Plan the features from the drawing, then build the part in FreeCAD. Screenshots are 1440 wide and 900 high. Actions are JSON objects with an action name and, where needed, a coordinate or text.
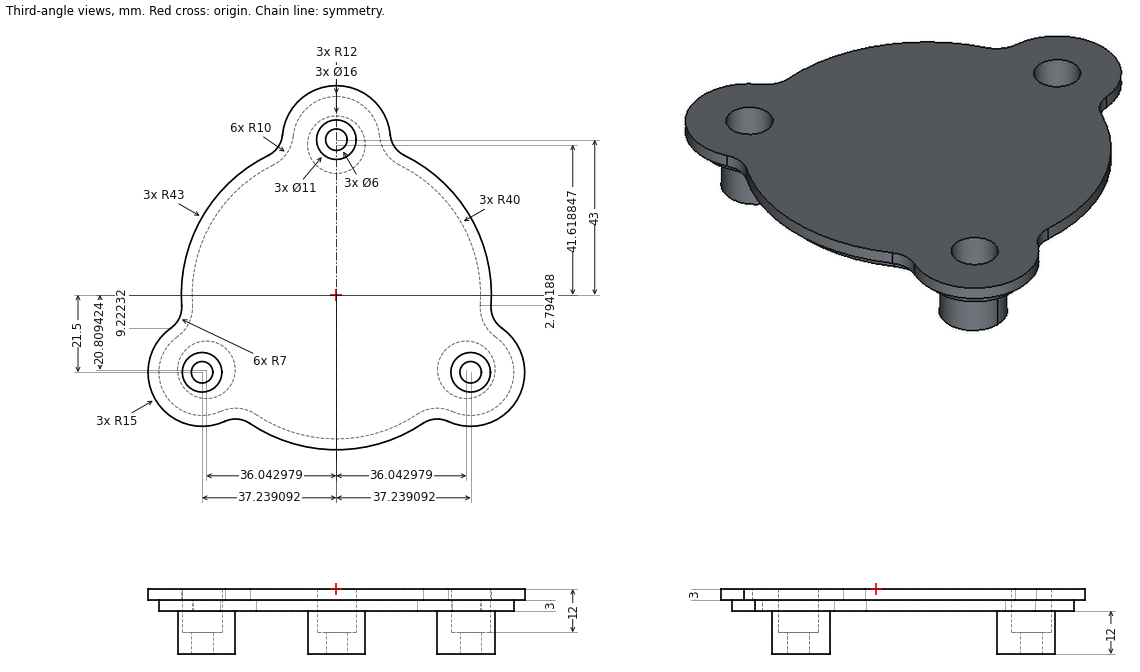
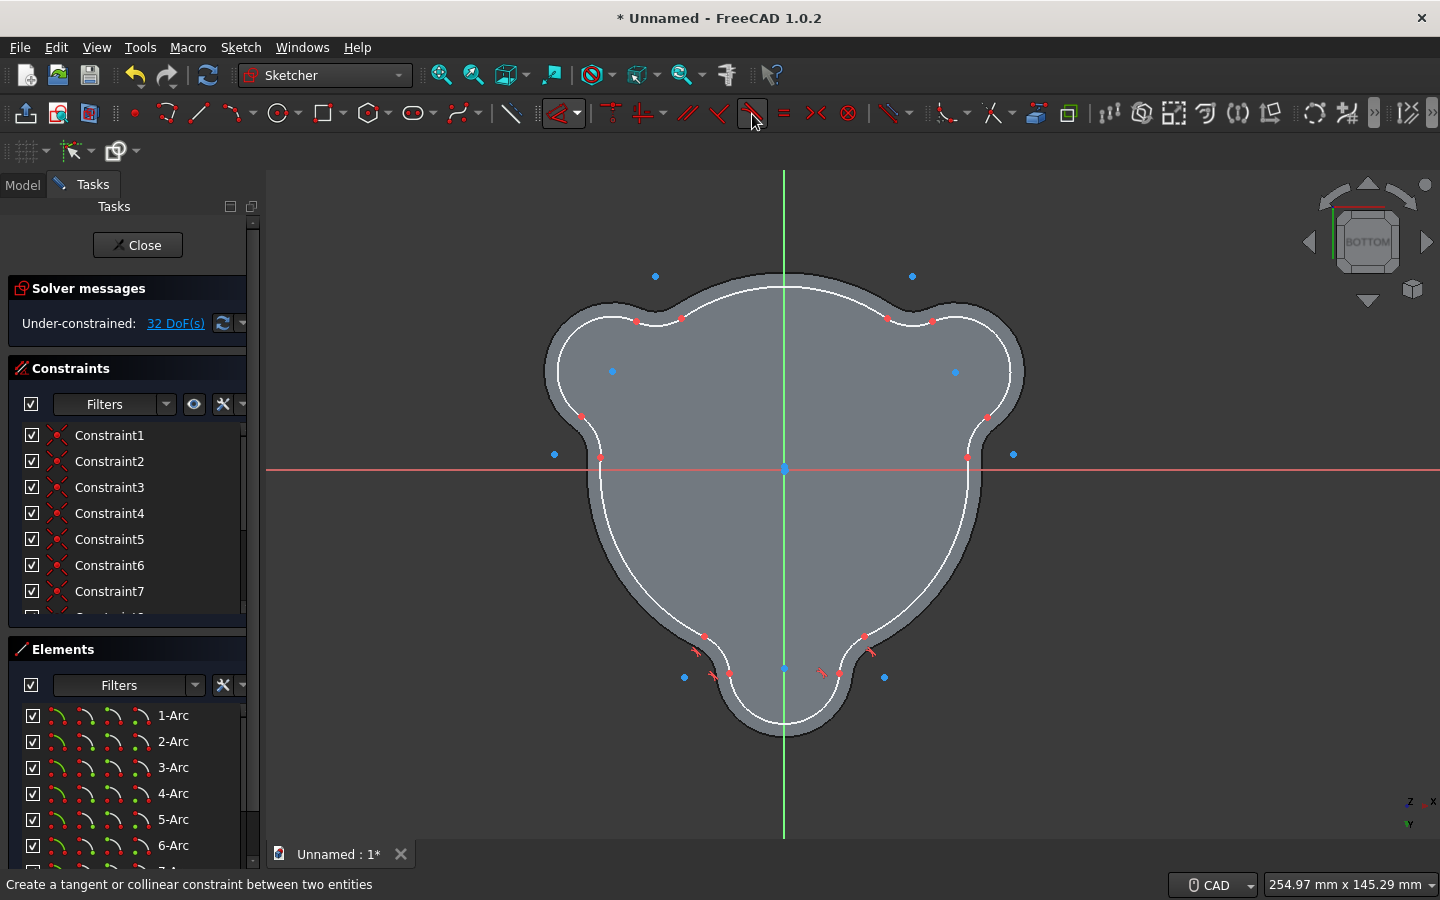
{"action": "left_click", "coordinate": [918, 598]}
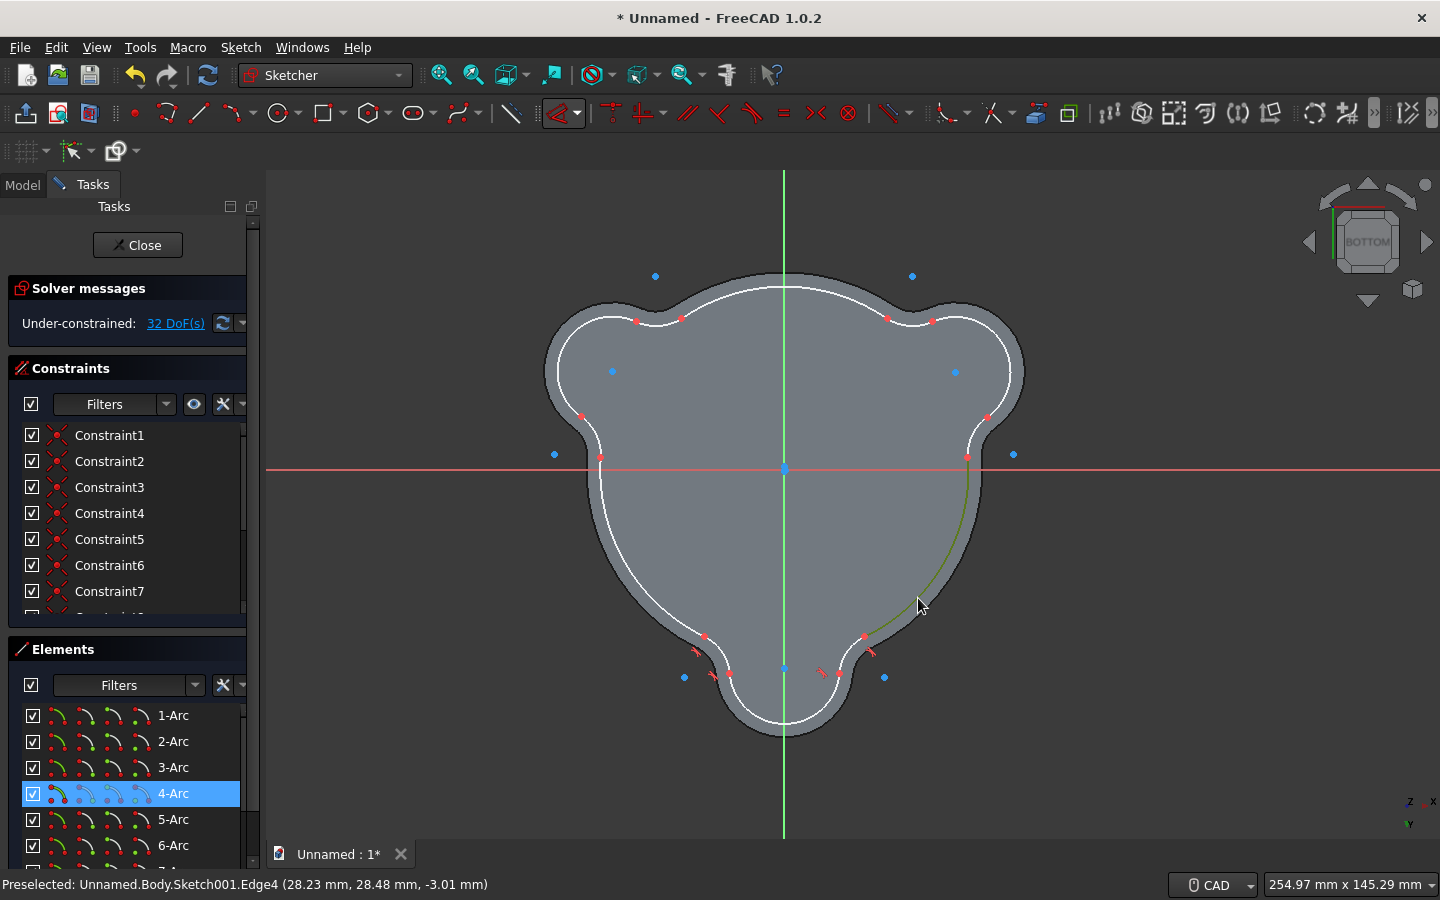
{"action": "left_click", "coordinate": [977, 427]}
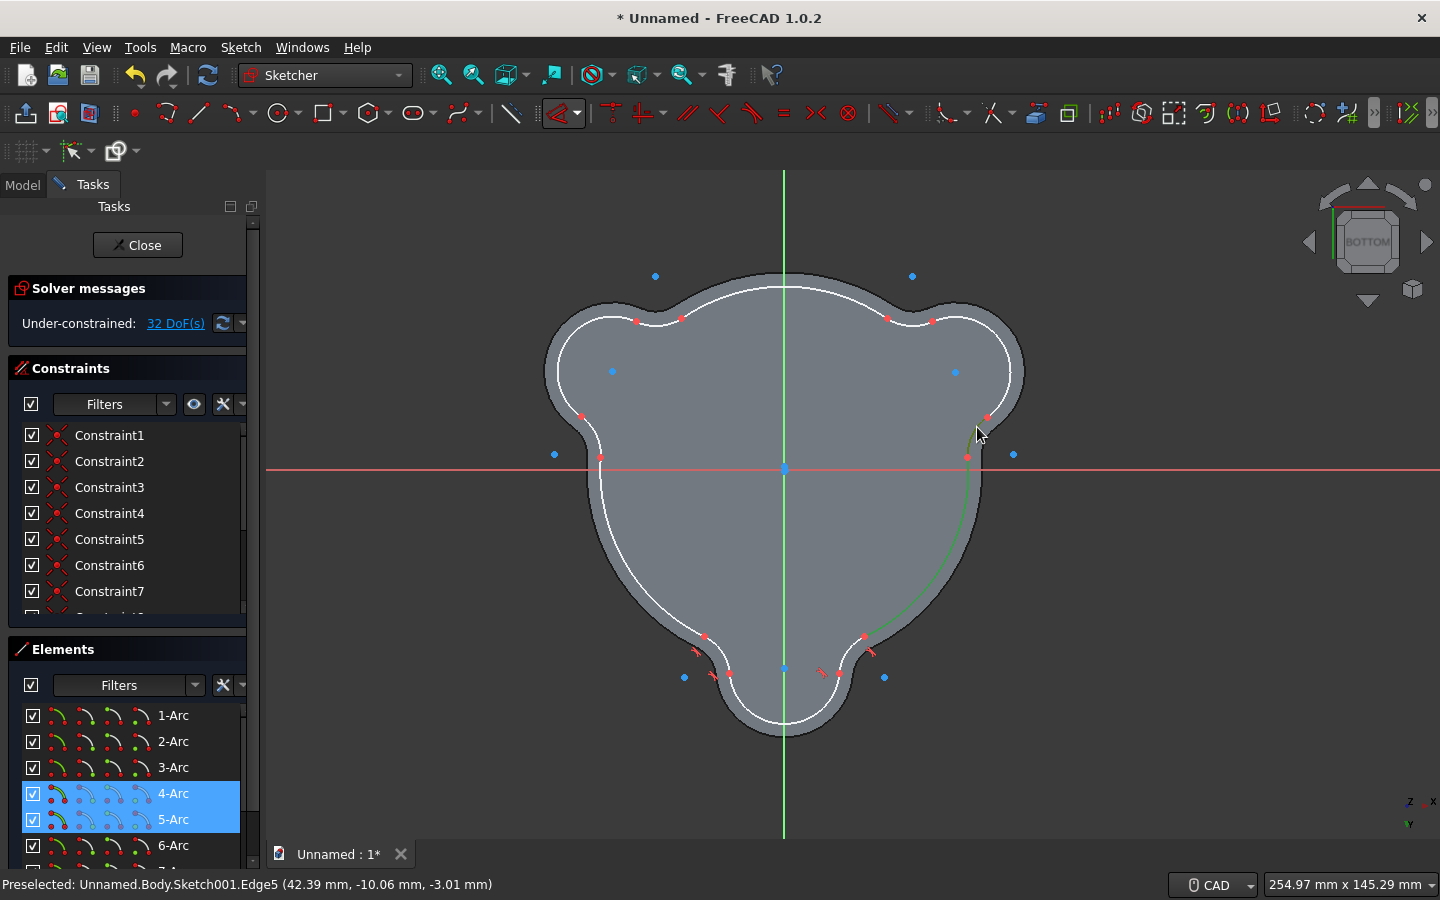
{"action": "left_click", "coordinate": [752, 114]}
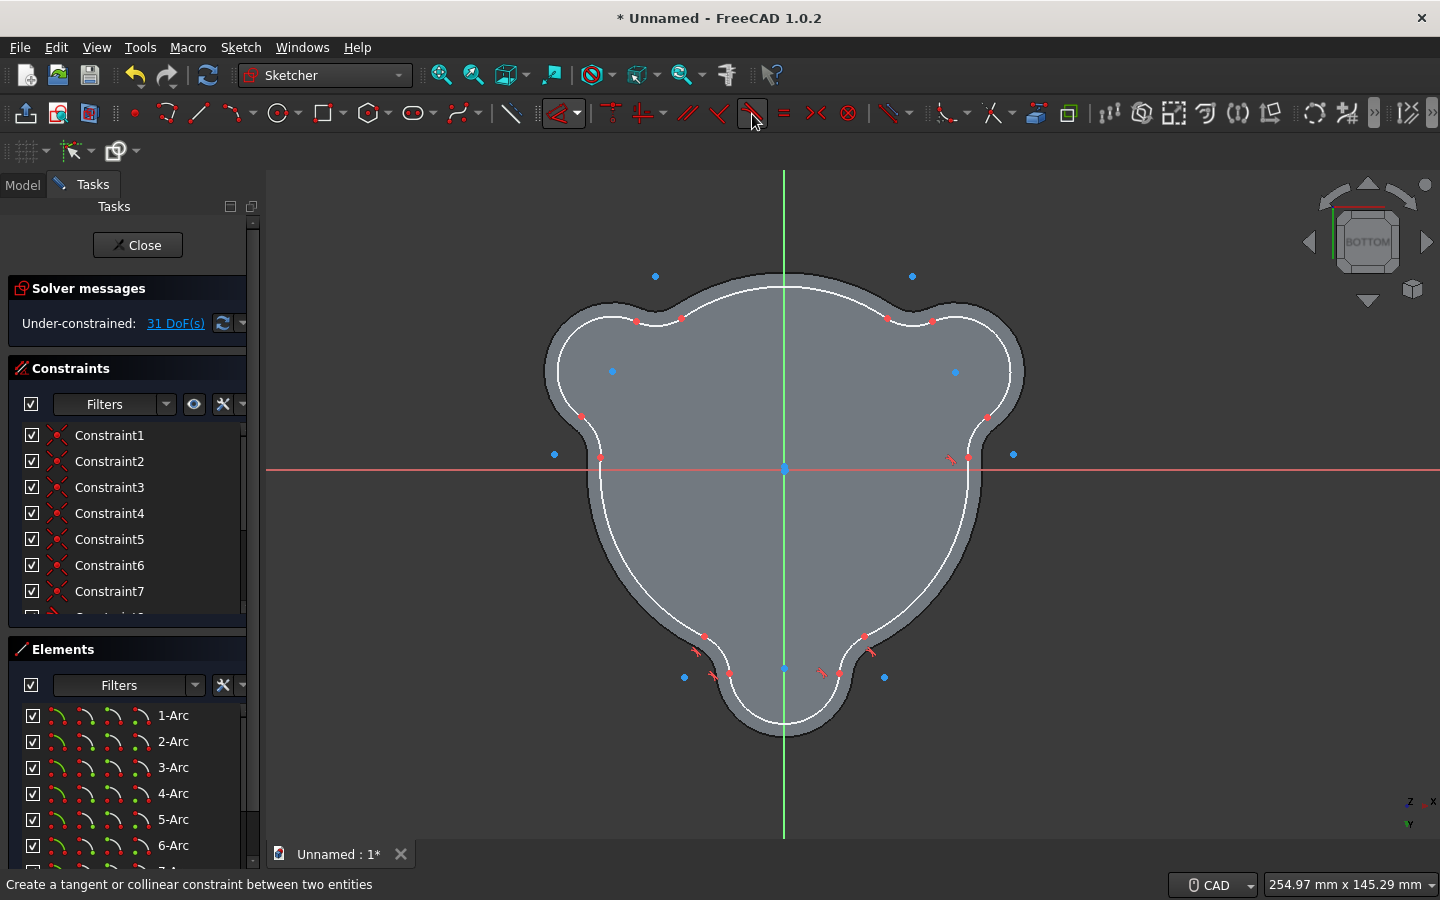
{"action": "left_click", "coordinate": [977, 427]}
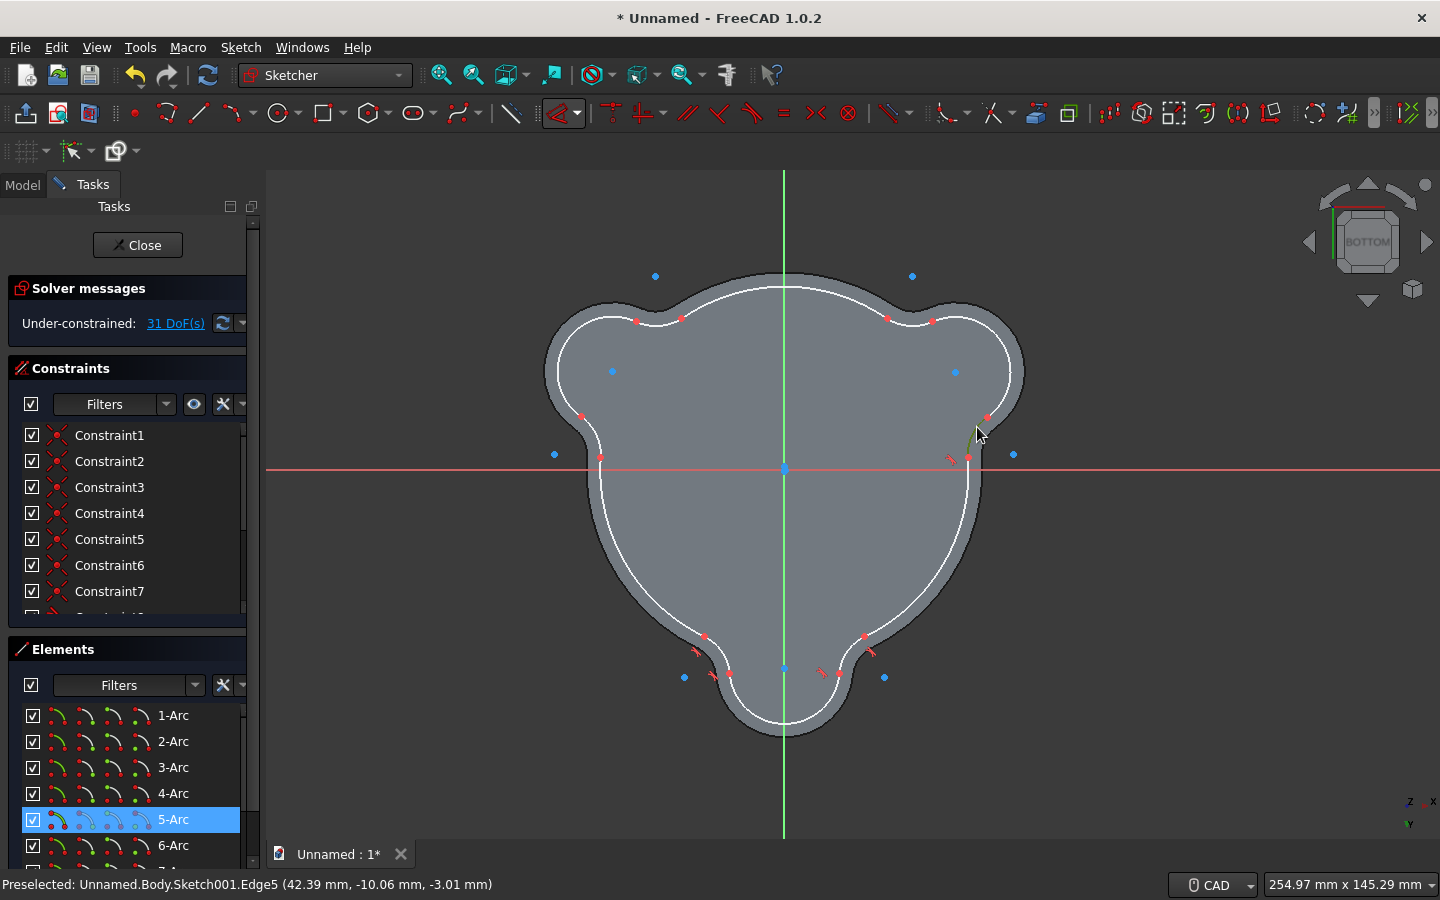
{"action": "left_click", "coordinate": [1010, 376]}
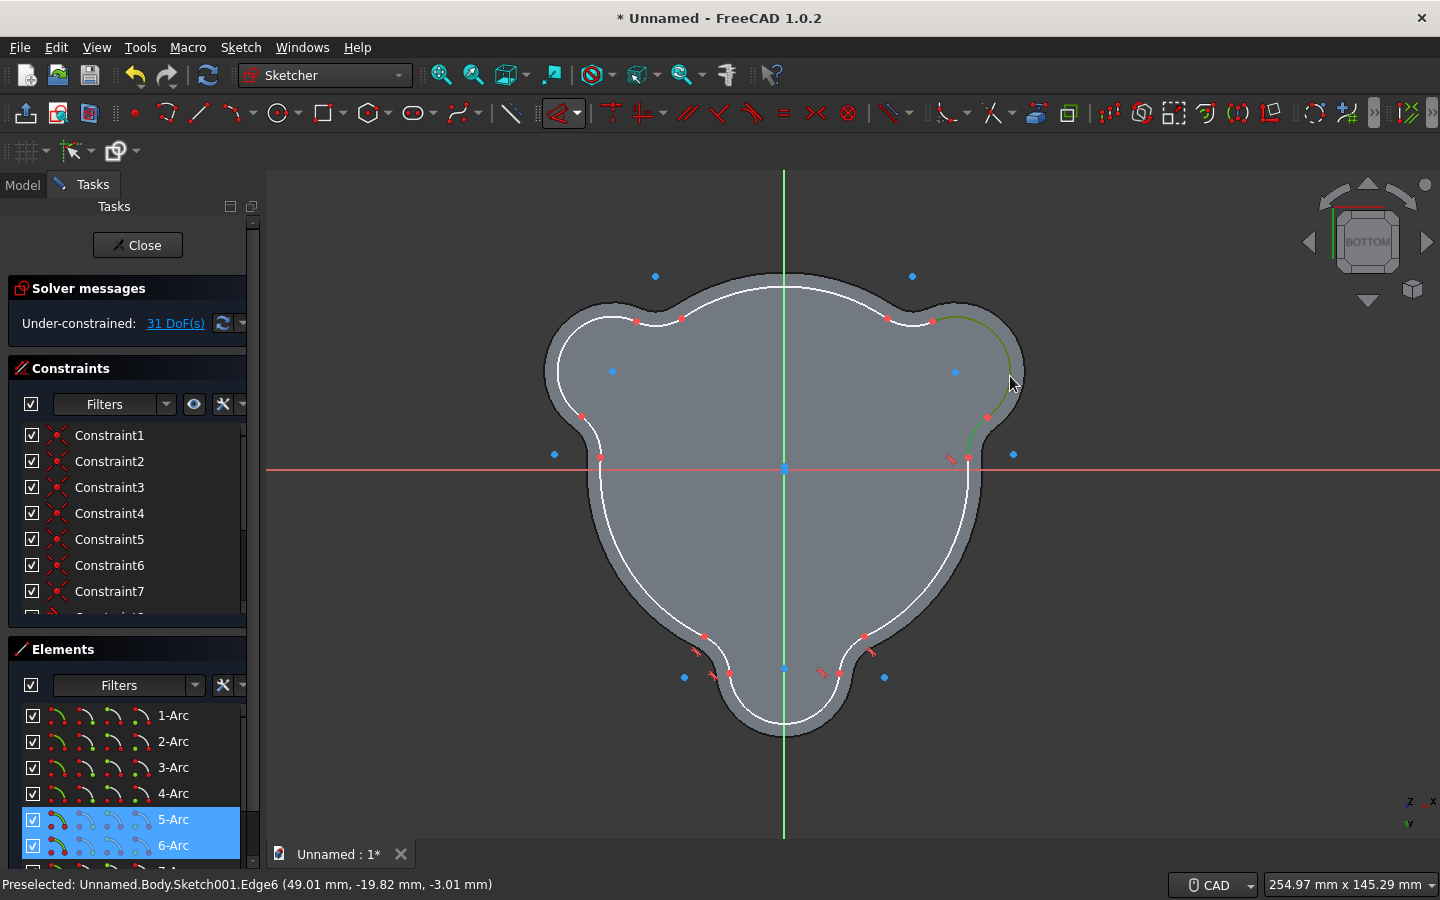
{"action": "left_click", "coordinate": [752, 114]}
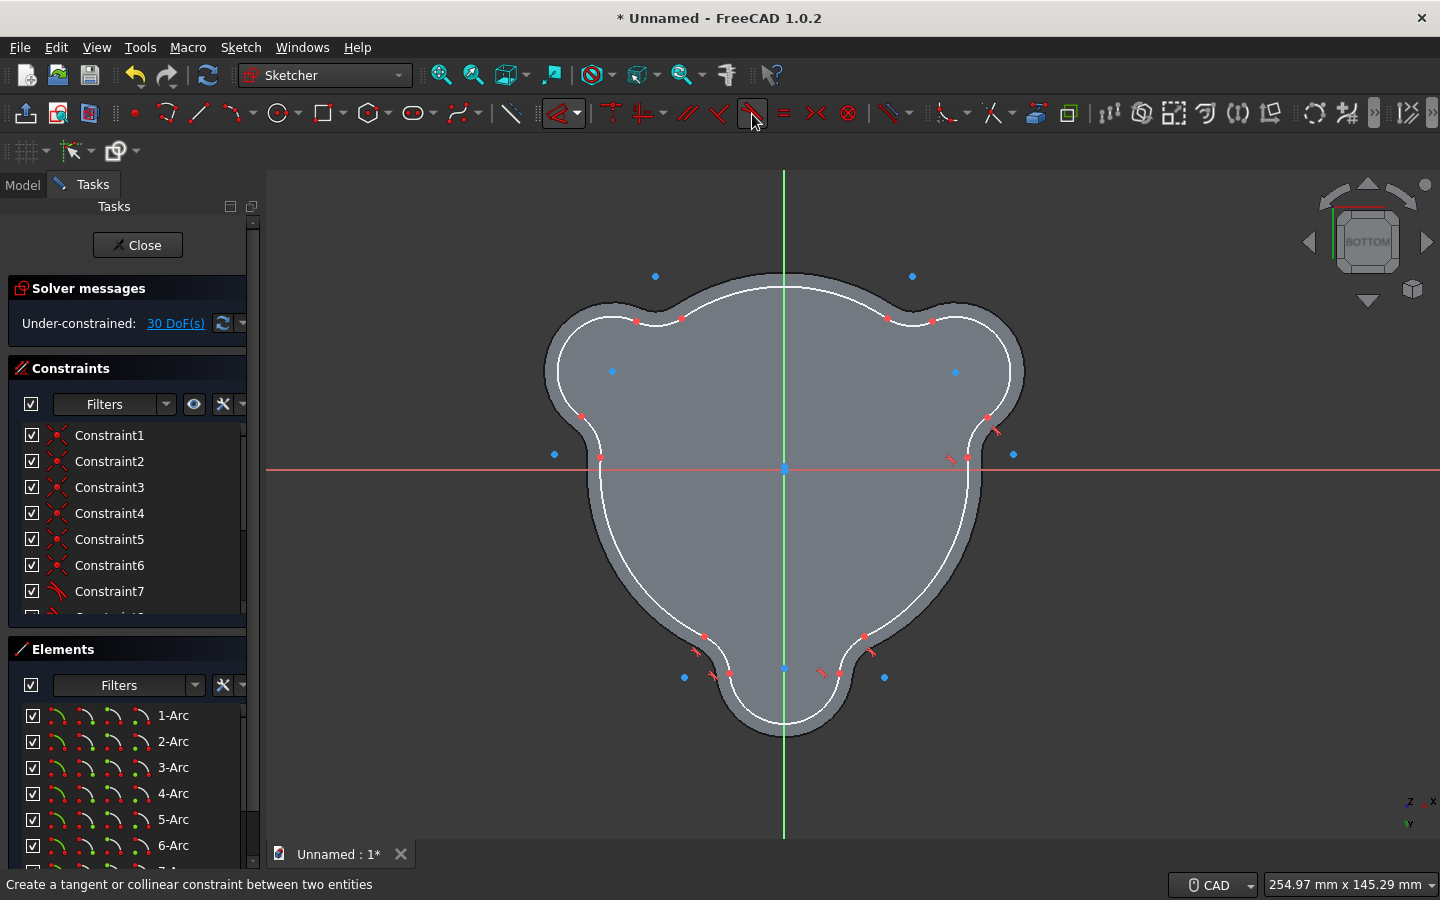
{"action": "left_click", "coordinate": [1010, 376]}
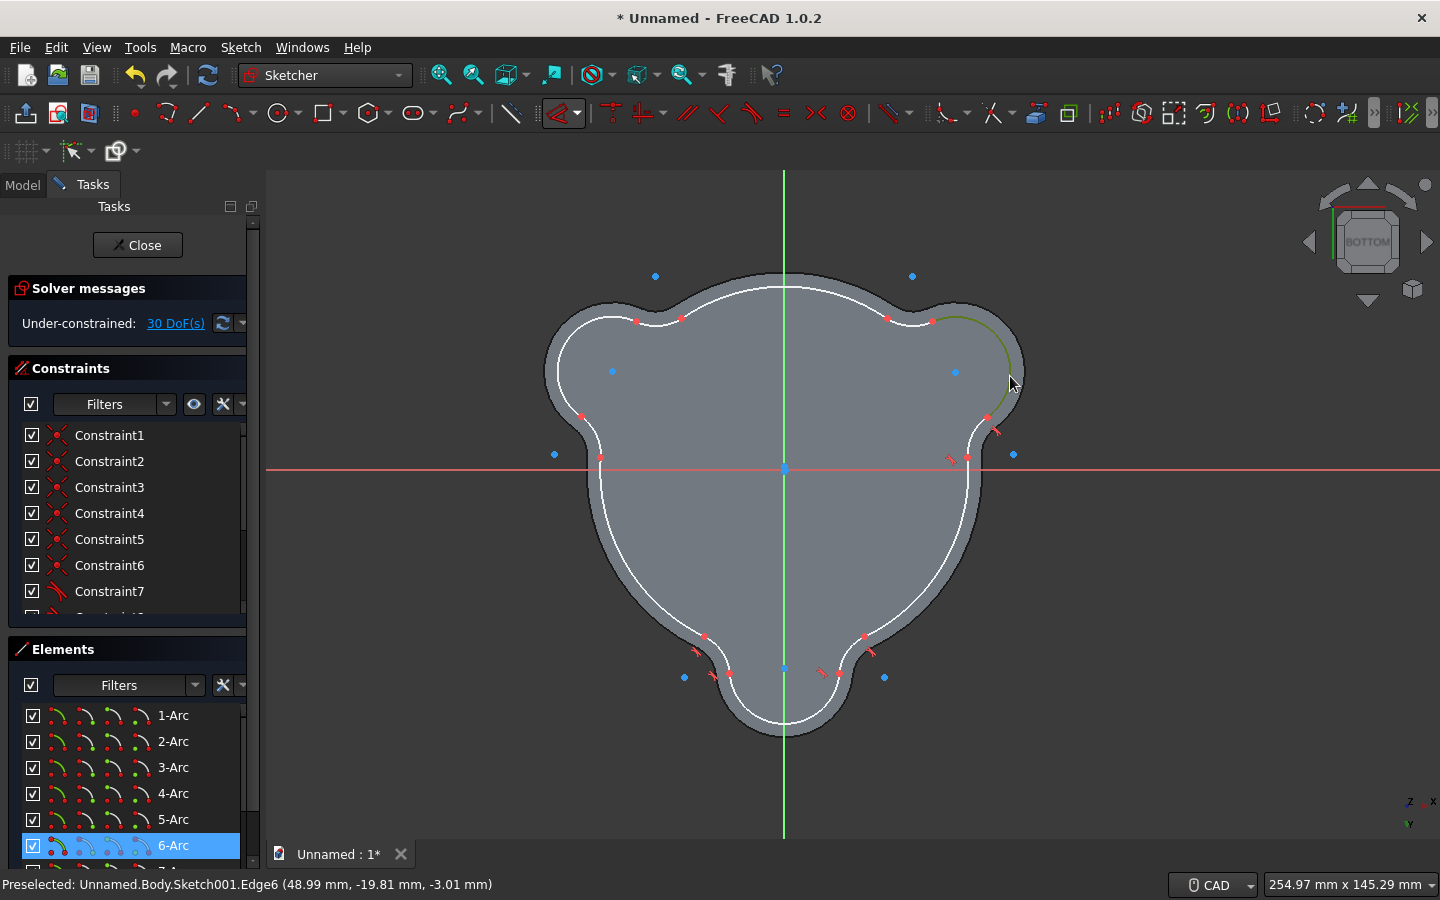
{"action": "left_click", "coordinate": [900, 324]}